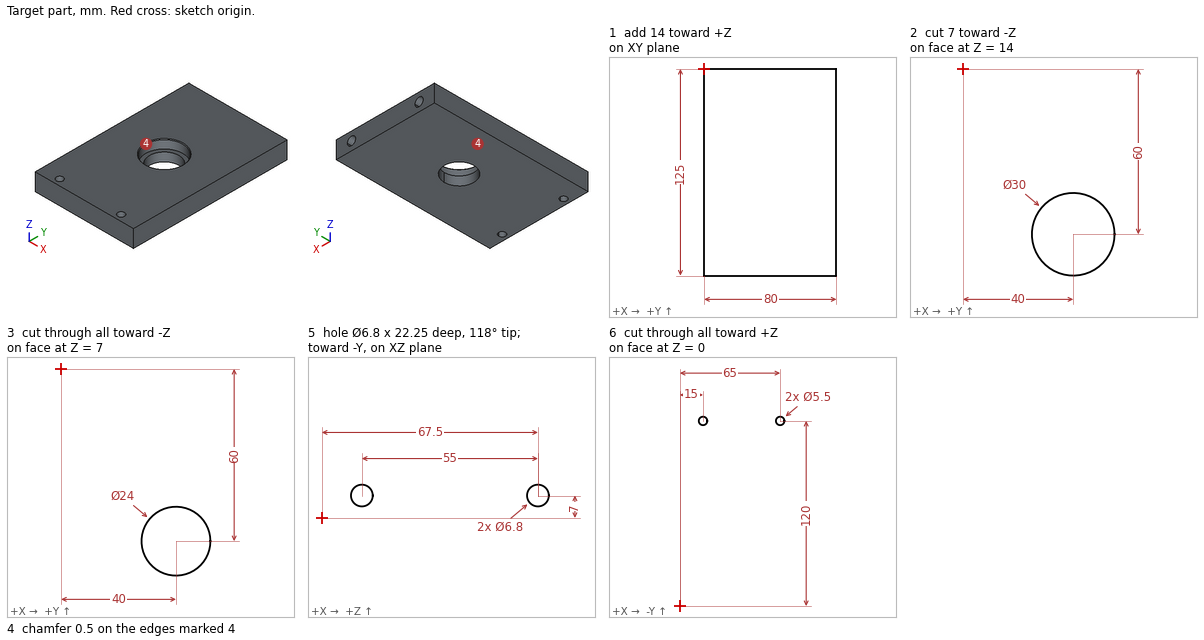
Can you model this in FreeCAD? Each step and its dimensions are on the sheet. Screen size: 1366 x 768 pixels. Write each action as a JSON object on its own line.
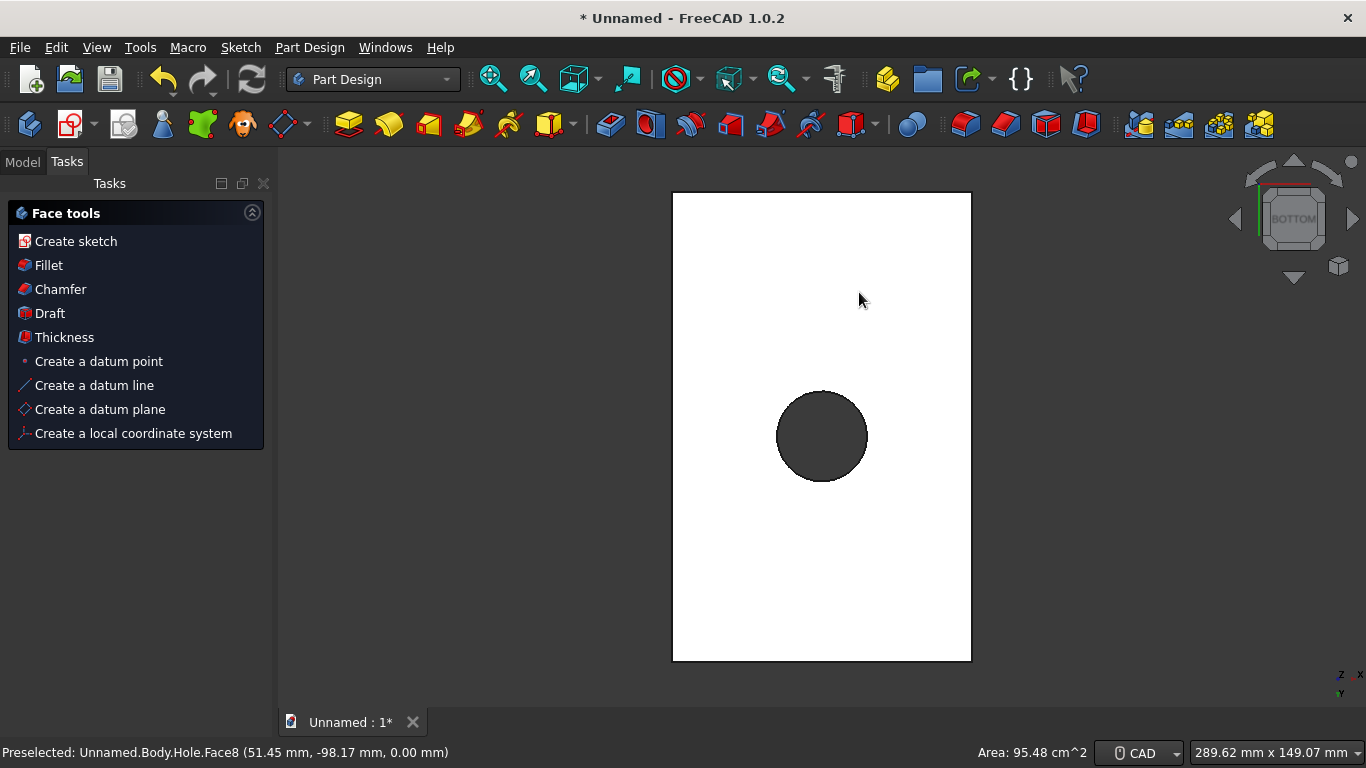
{"action": "left_click", "coordinate": [70, 124]}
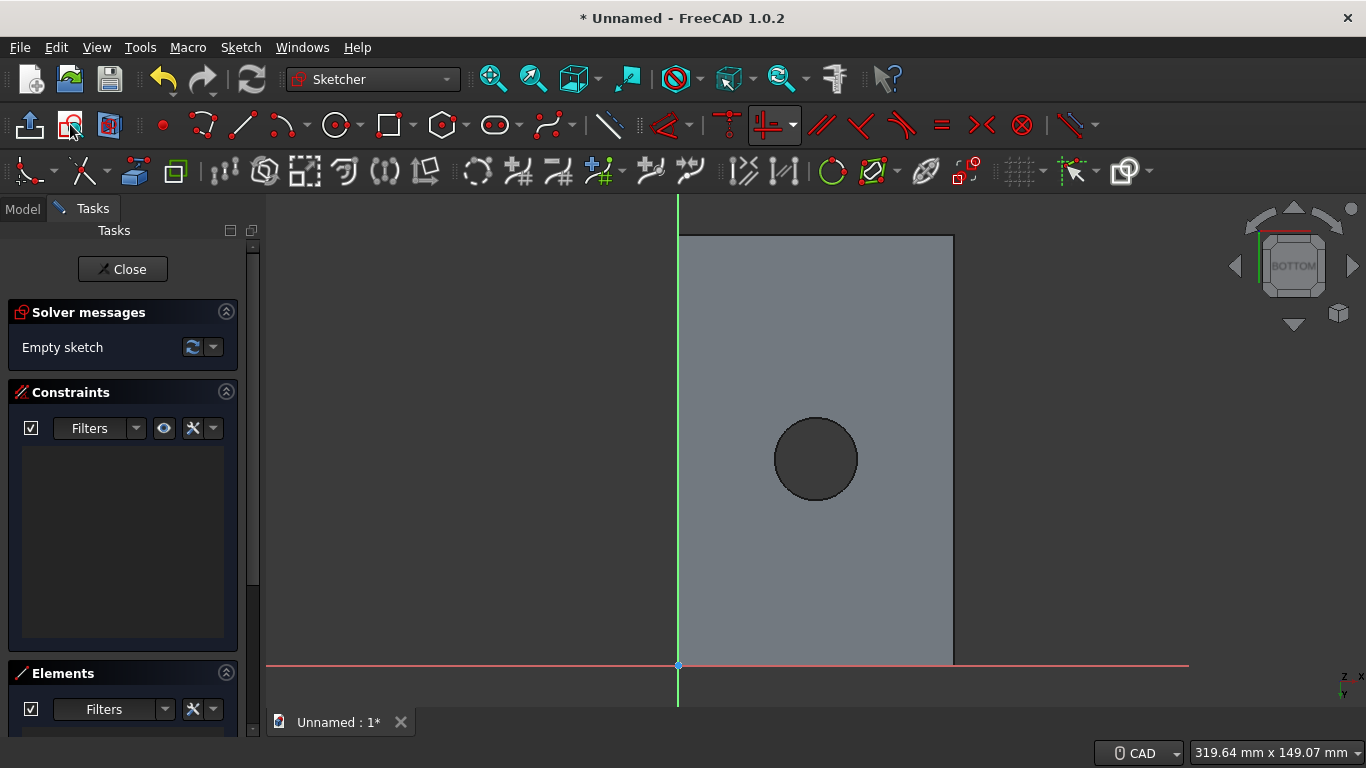
{"action": "scroll", "coordinate": [533, 433], "scroll_direction": "down", "scroll_amount": 1}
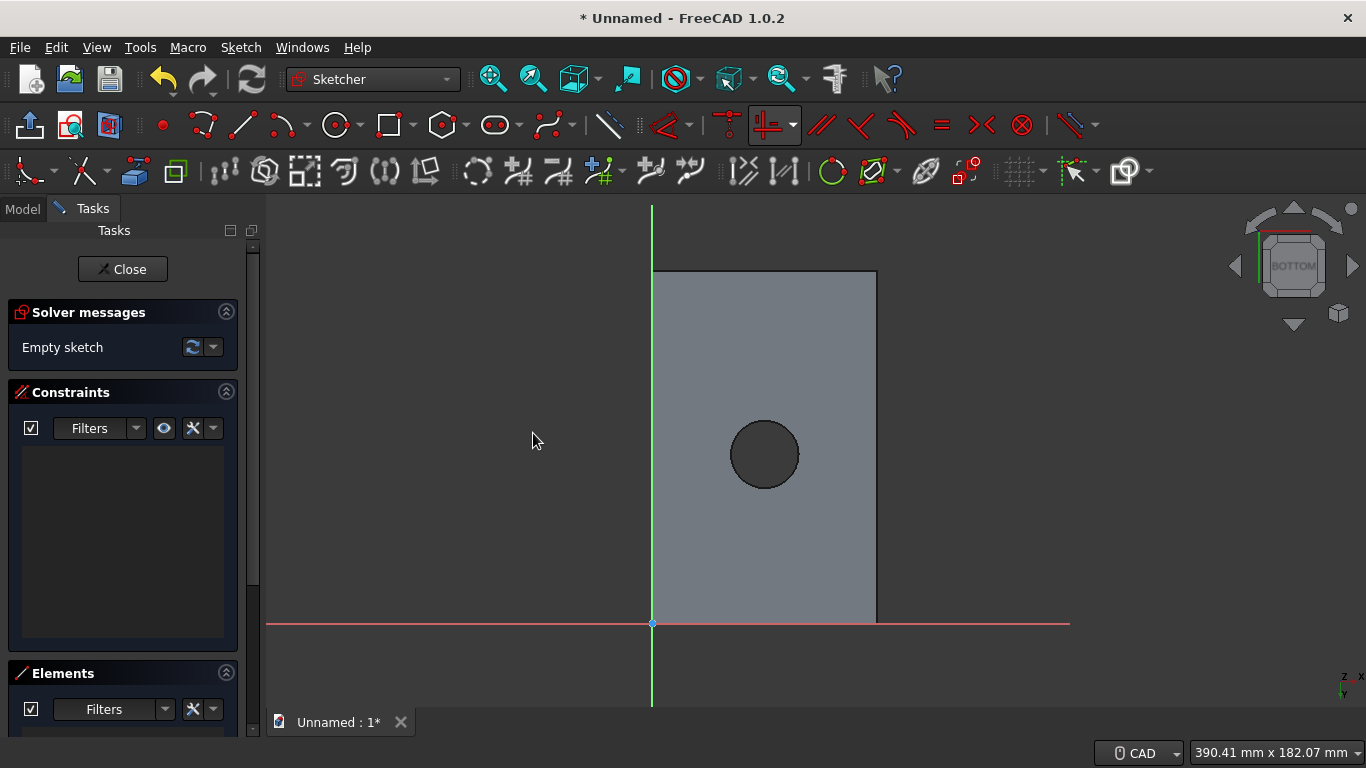
{"action": "left_click", "coordinate": [336, 126]}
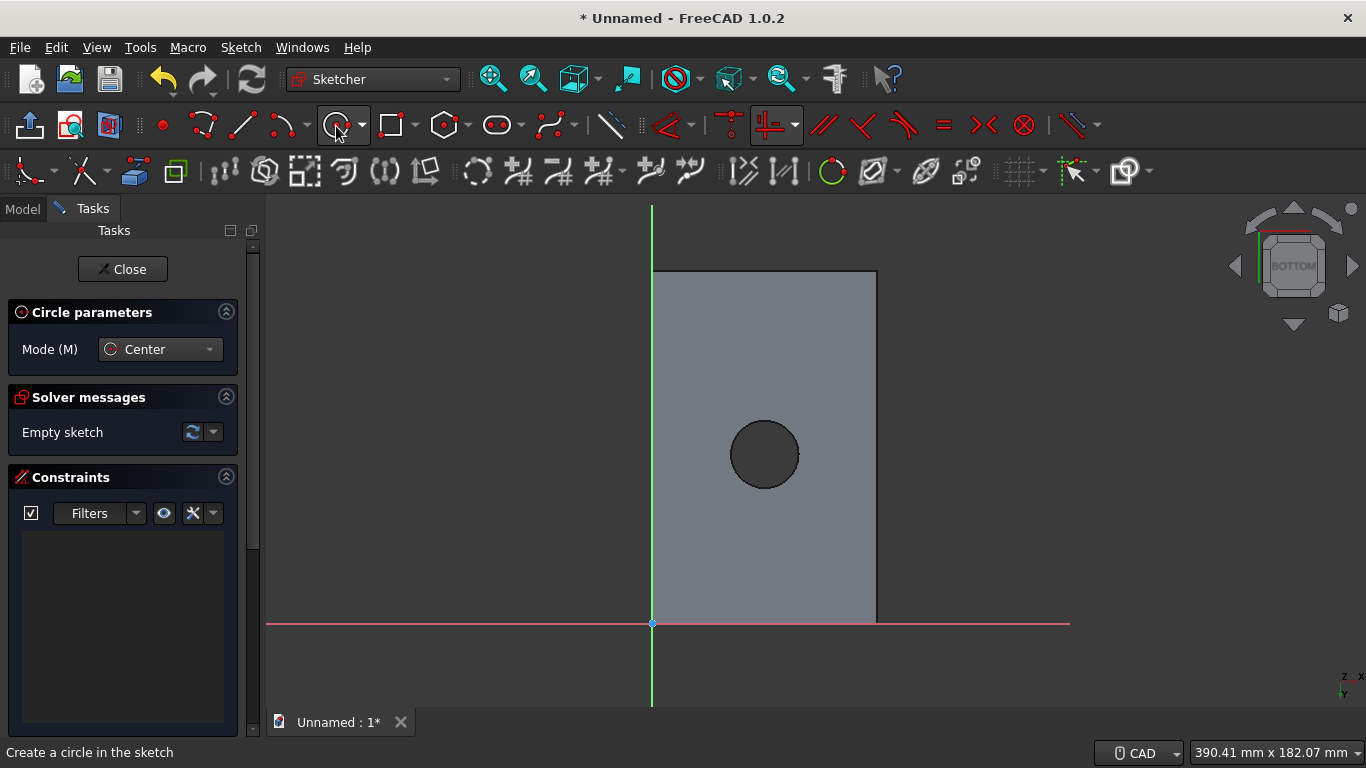
{"action": "scroll", "coordinate": [835, 285], "scroll_direction": "up", "scroll_amount": 6}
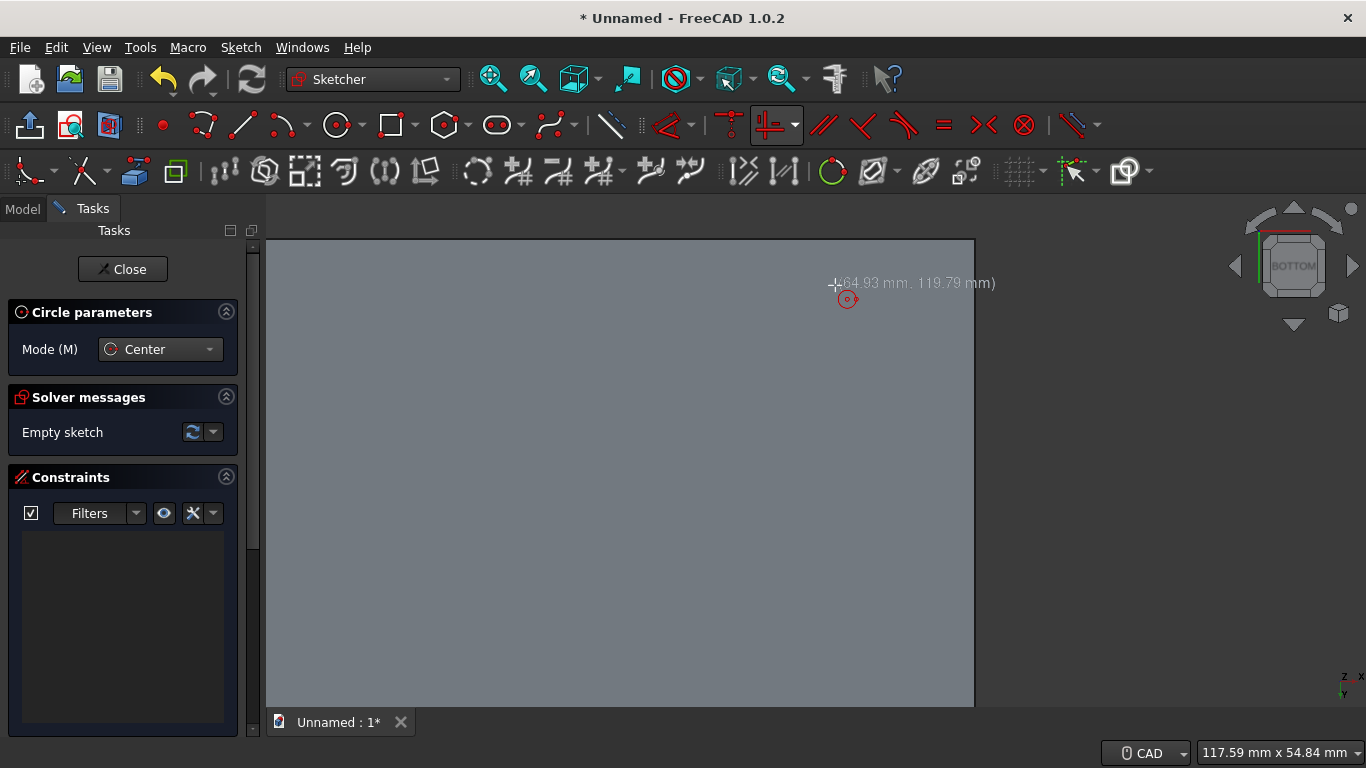
{"action": "left_click", "coordinate": [834, 286]}
{"action": "left_click", "coordinate": [853, 268]}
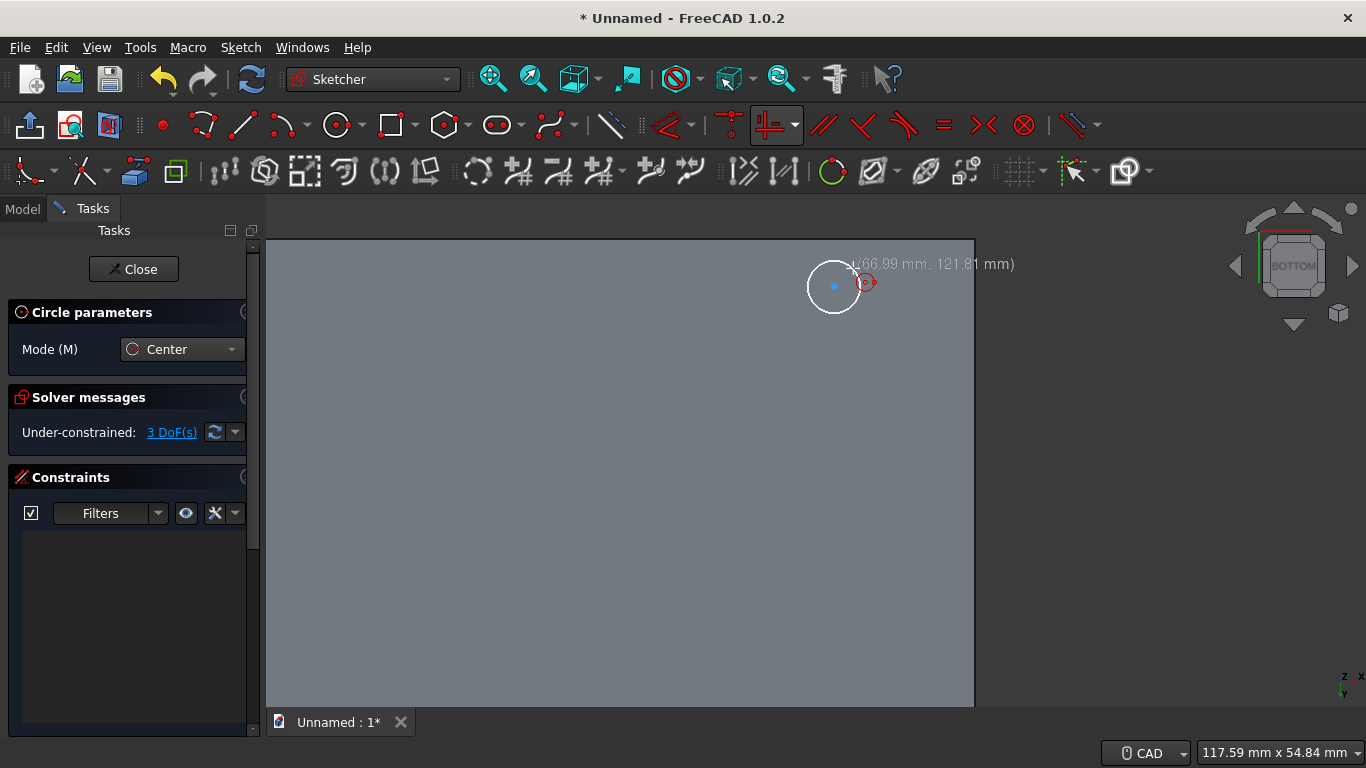
{"action": "left_click", "coordinate": [367, 286]}
{"action": "left_click", "coordinate": [385, 268]}
{"action": "key", "text": "Escape"}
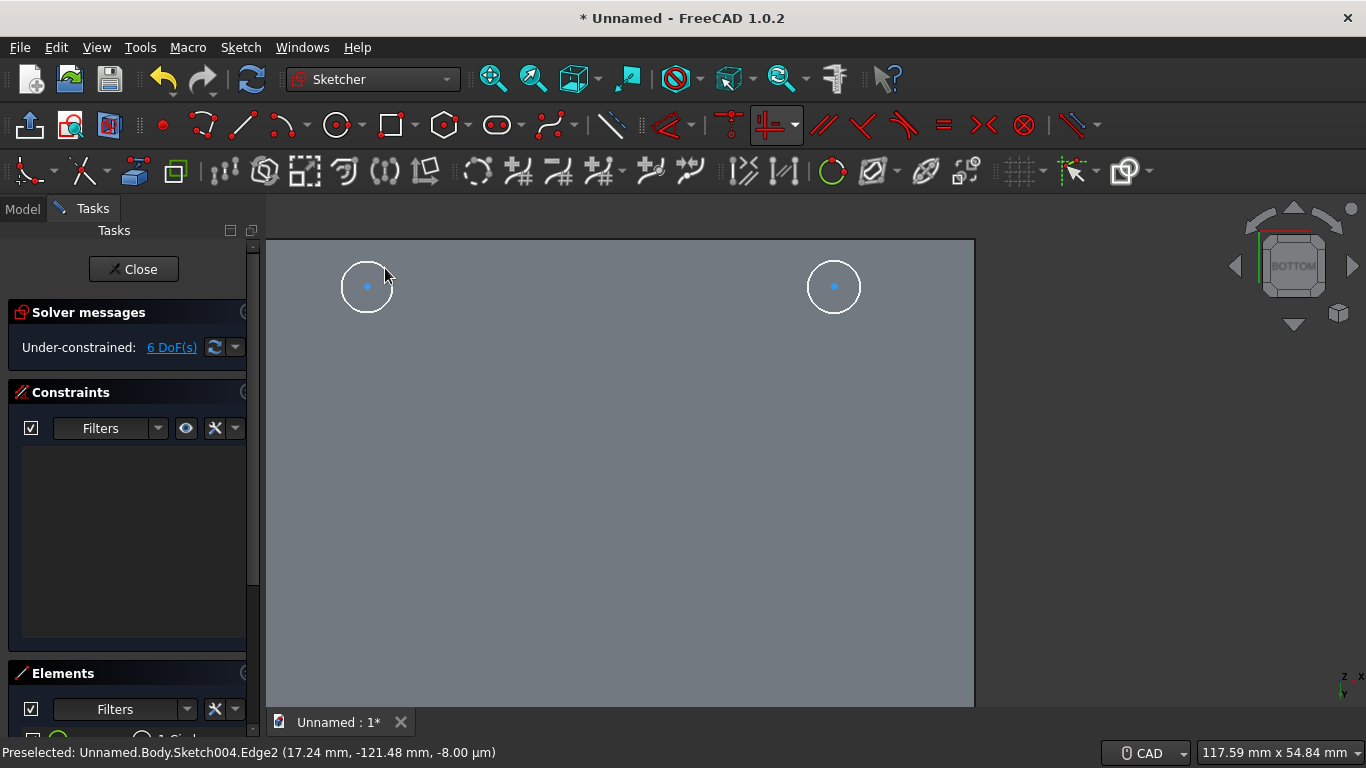
{"action": "left_click", "coordinate": [852, 268]}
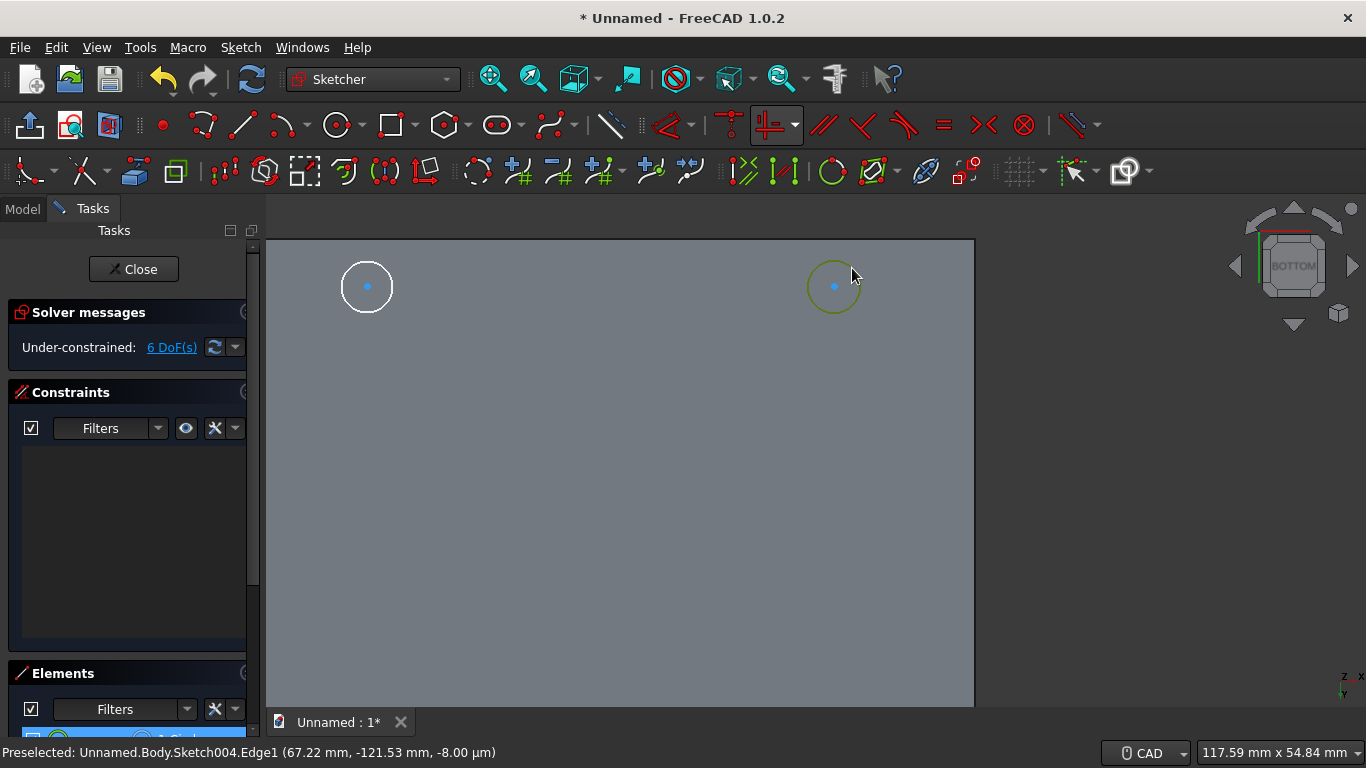
{"action": "left_click", "coordinate": [385, 269]}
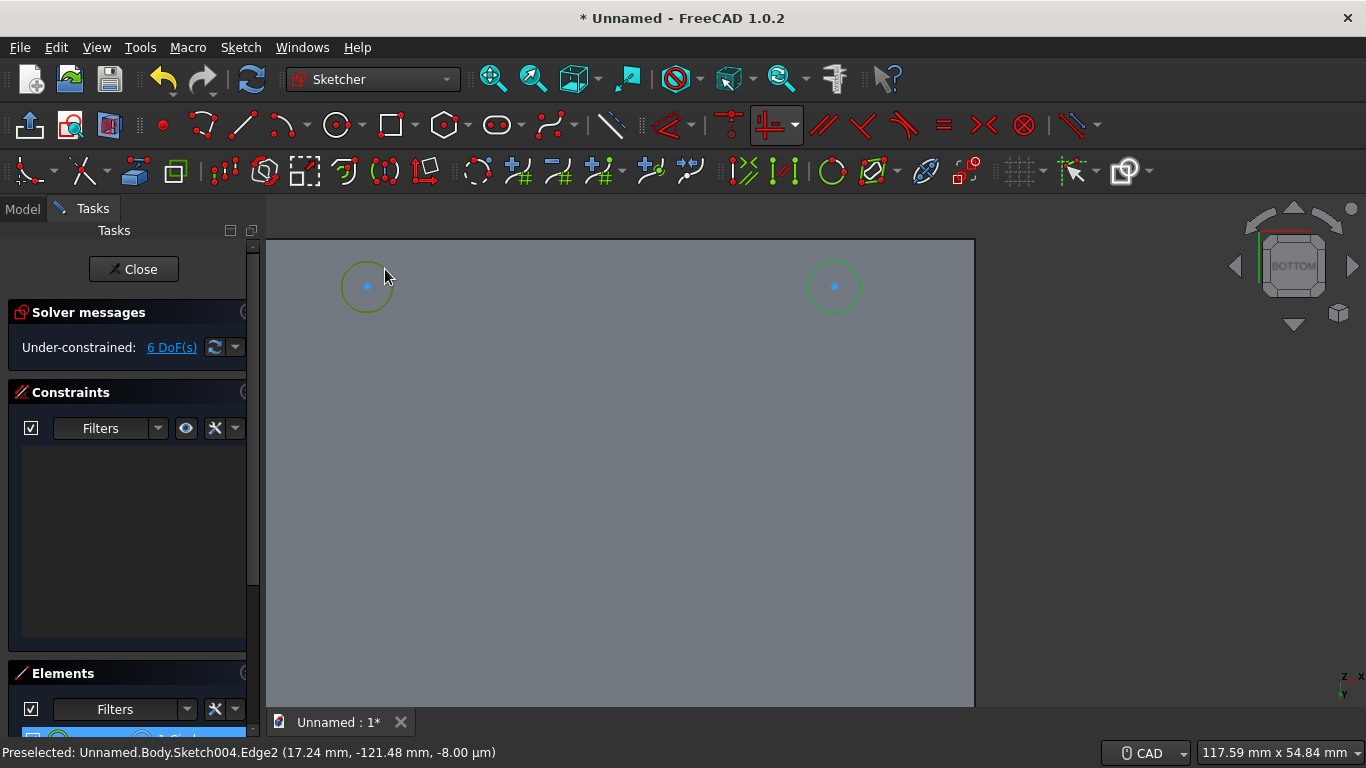
{"action": "key", "text": "e"}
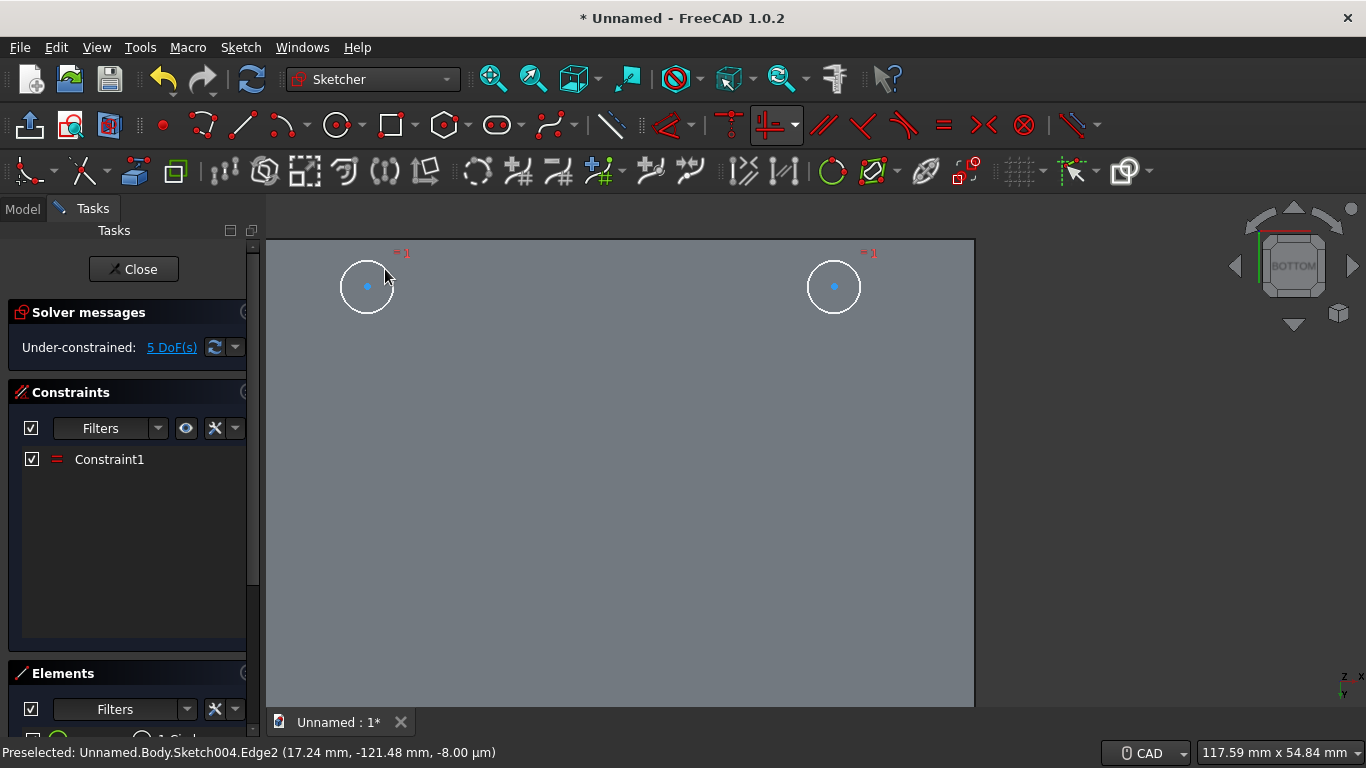
{"action": "left_click", "coordinate": [834, 287]}